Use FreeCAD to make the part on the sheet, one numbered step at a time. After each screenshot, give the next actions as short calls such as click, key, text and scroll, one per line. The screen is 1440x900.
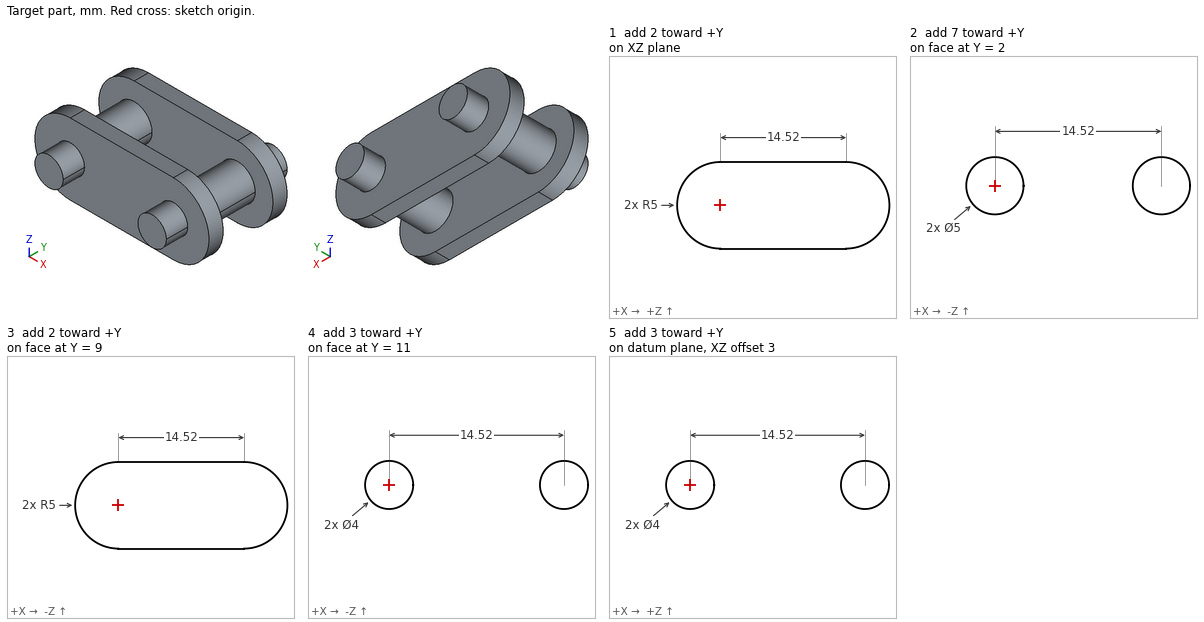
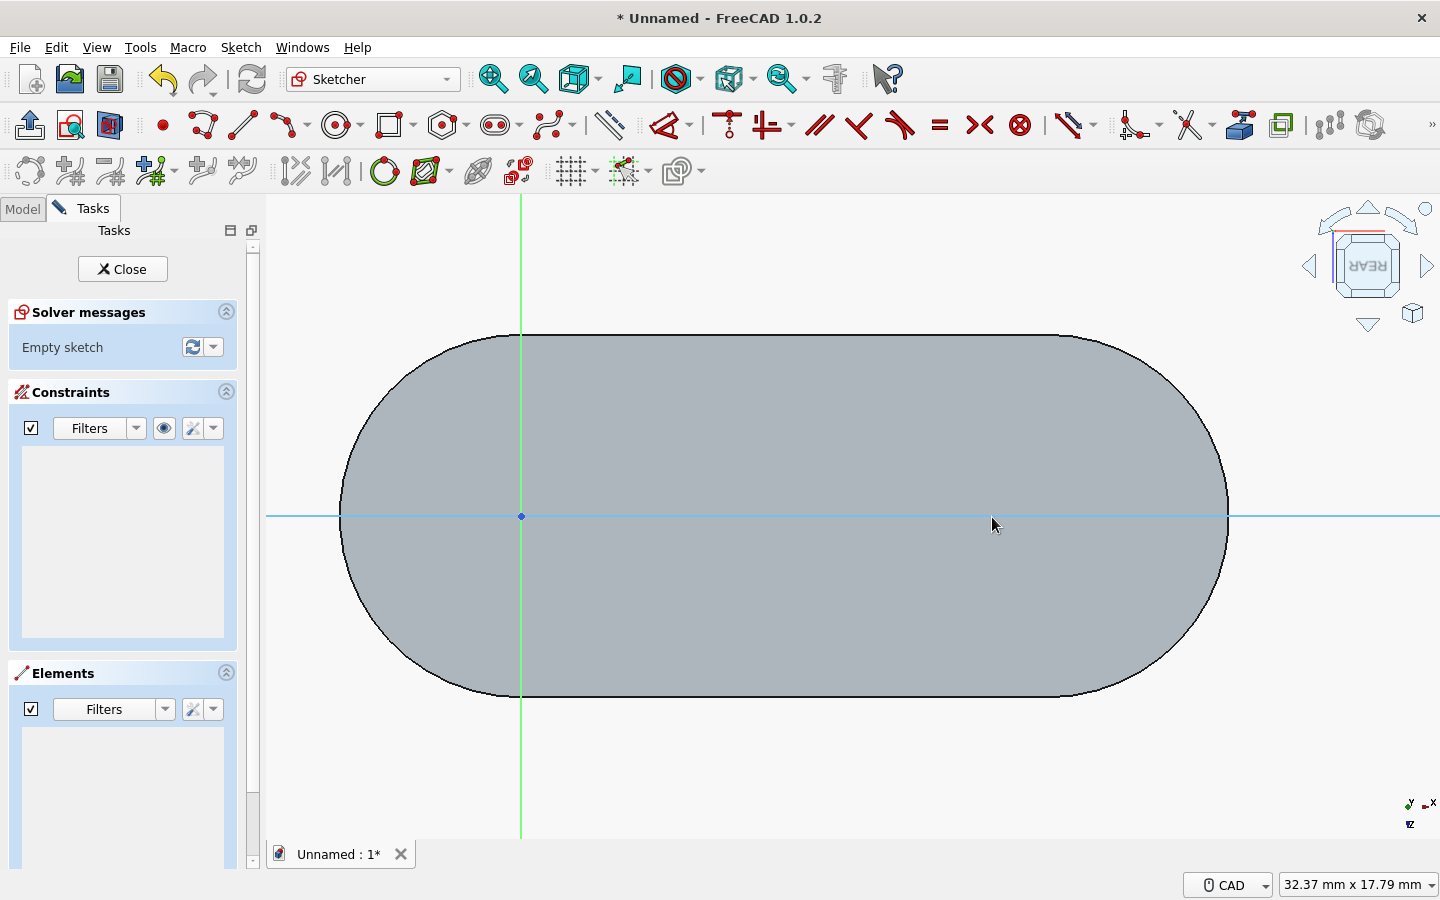
click(336, 126)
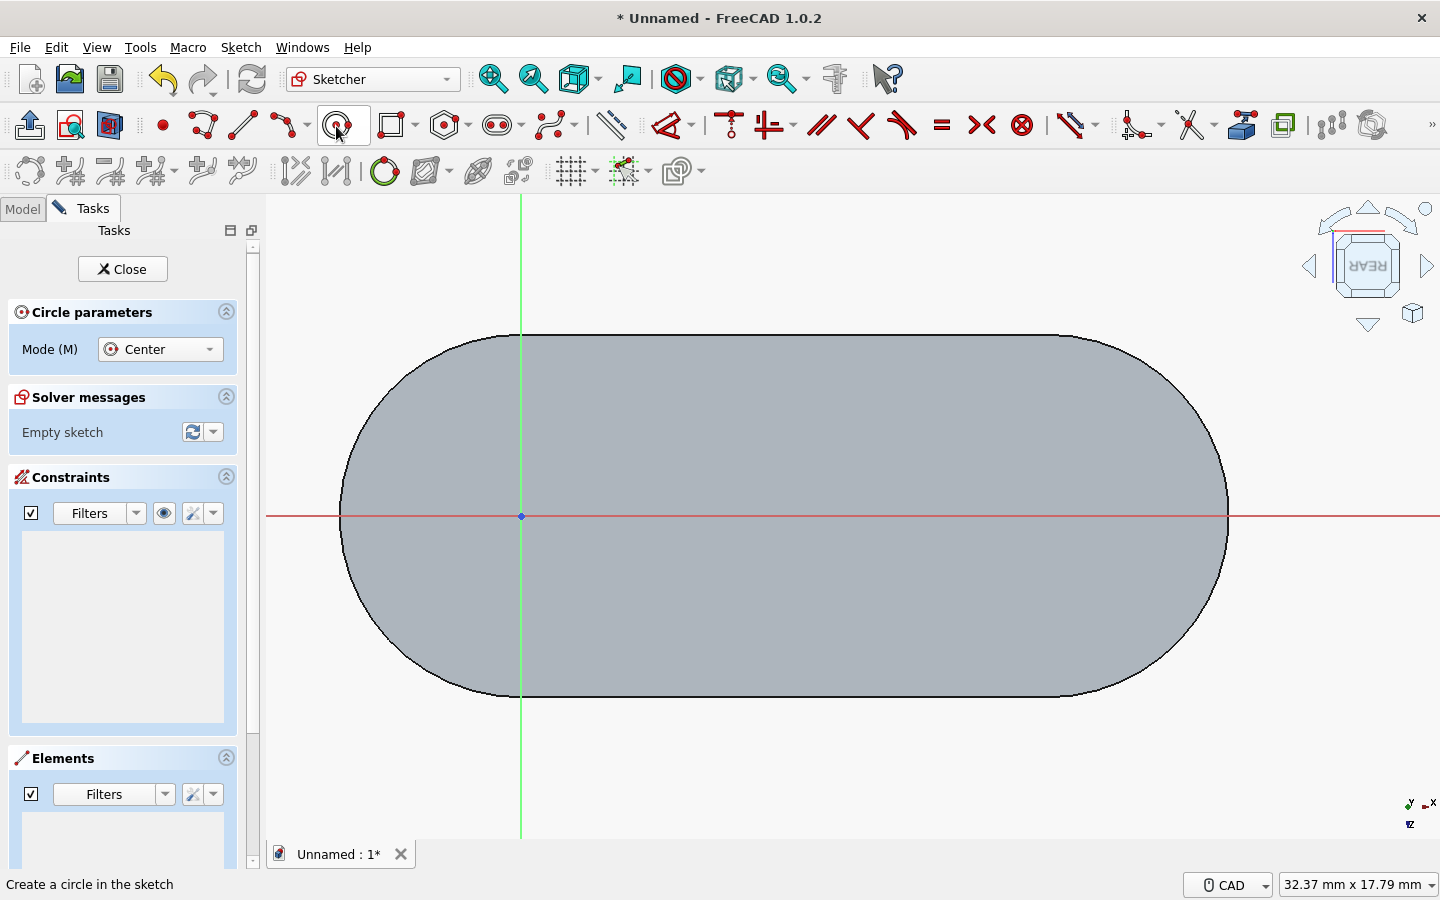
click(521, 516)
move(585, 452)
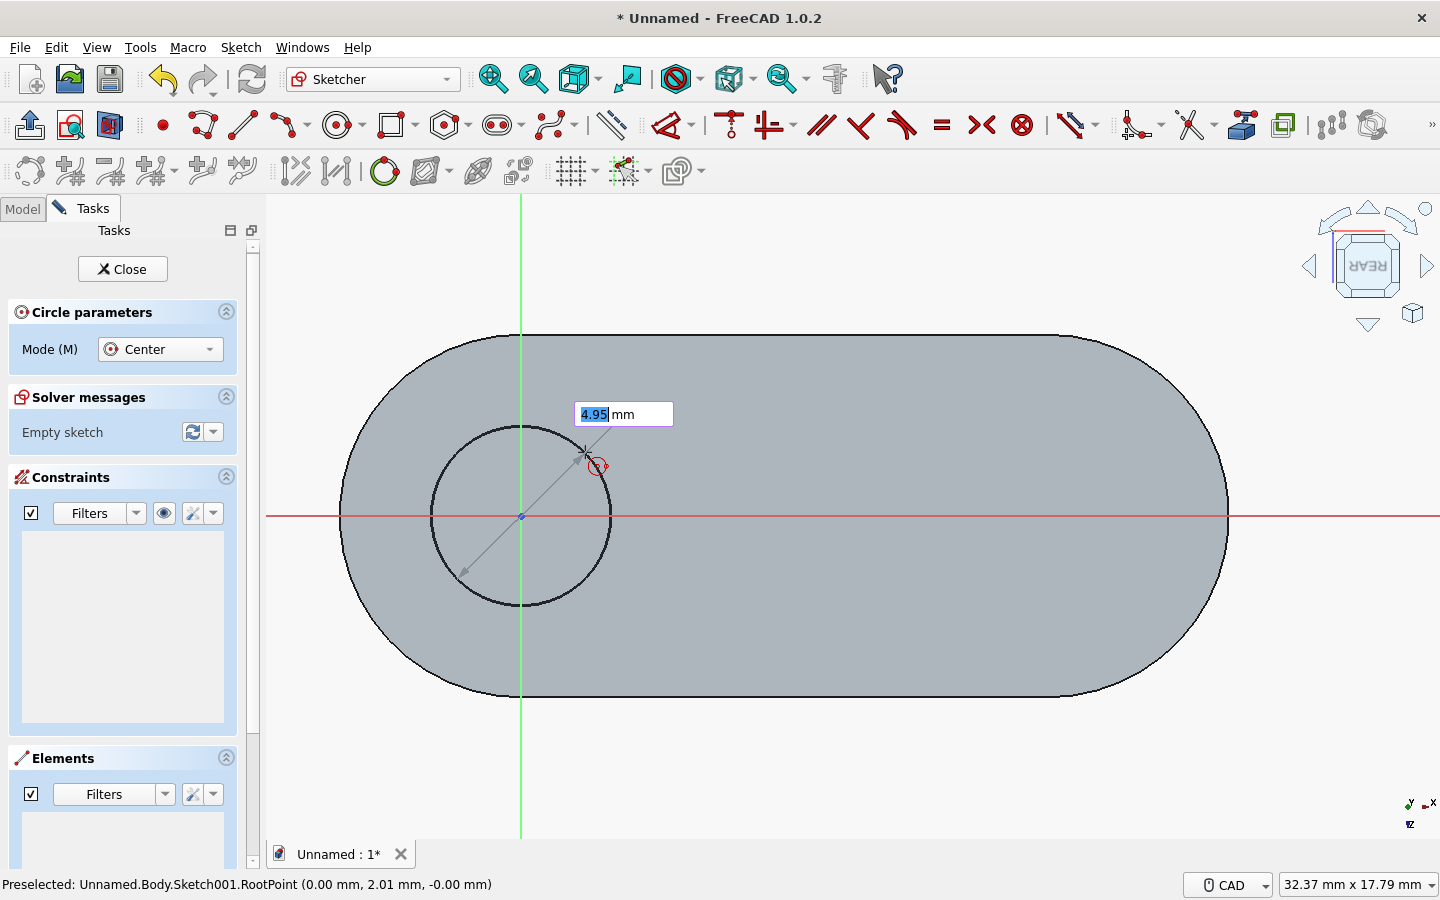
text(5)
key(Return)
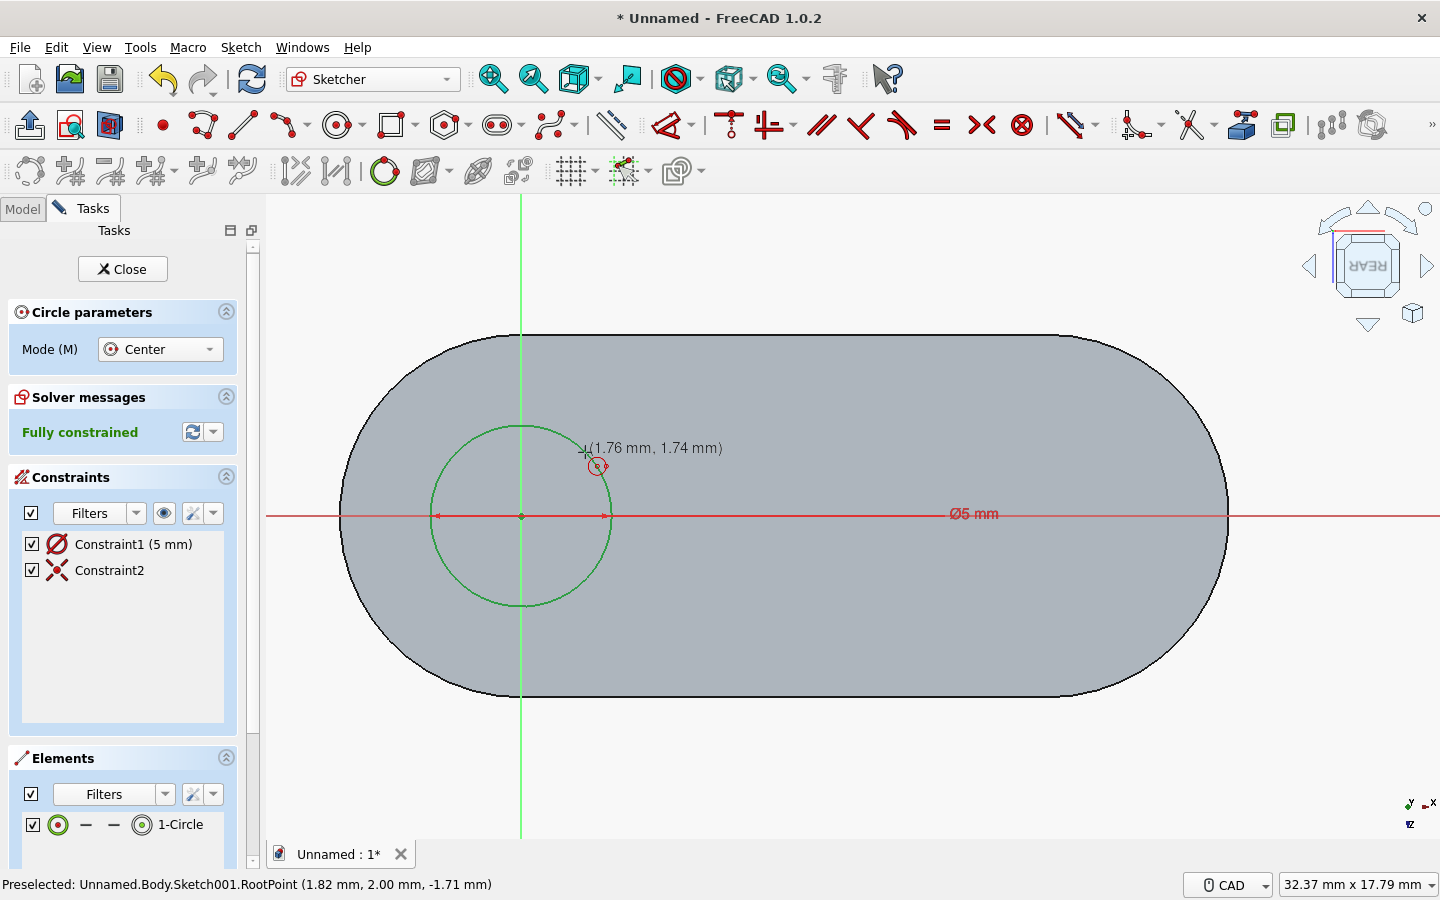
click(1048, 516)
move(1112, 452)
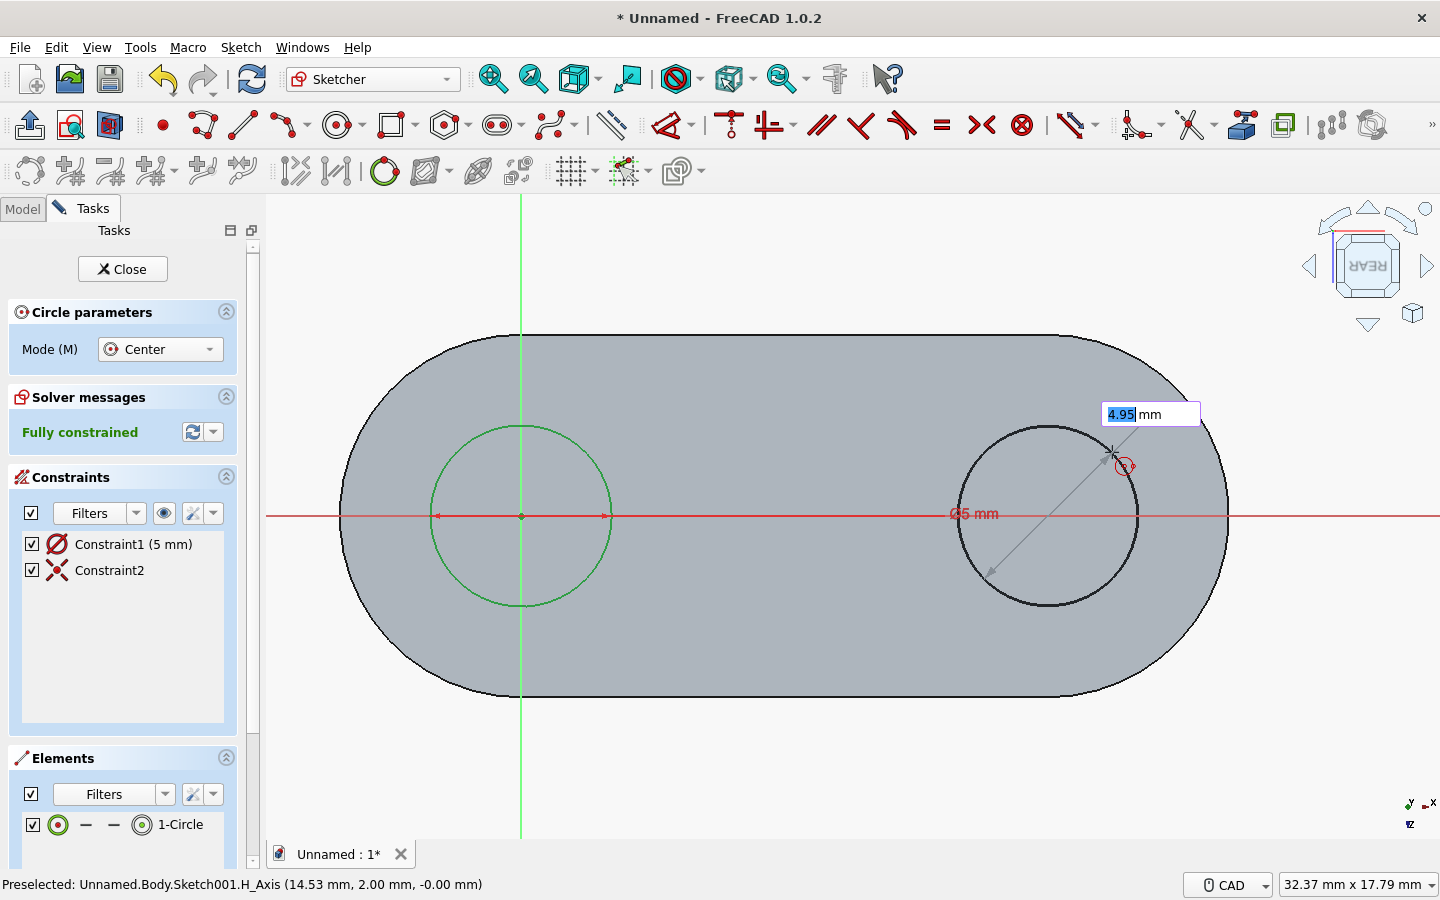
text(5)
key(Return)
key(Escape)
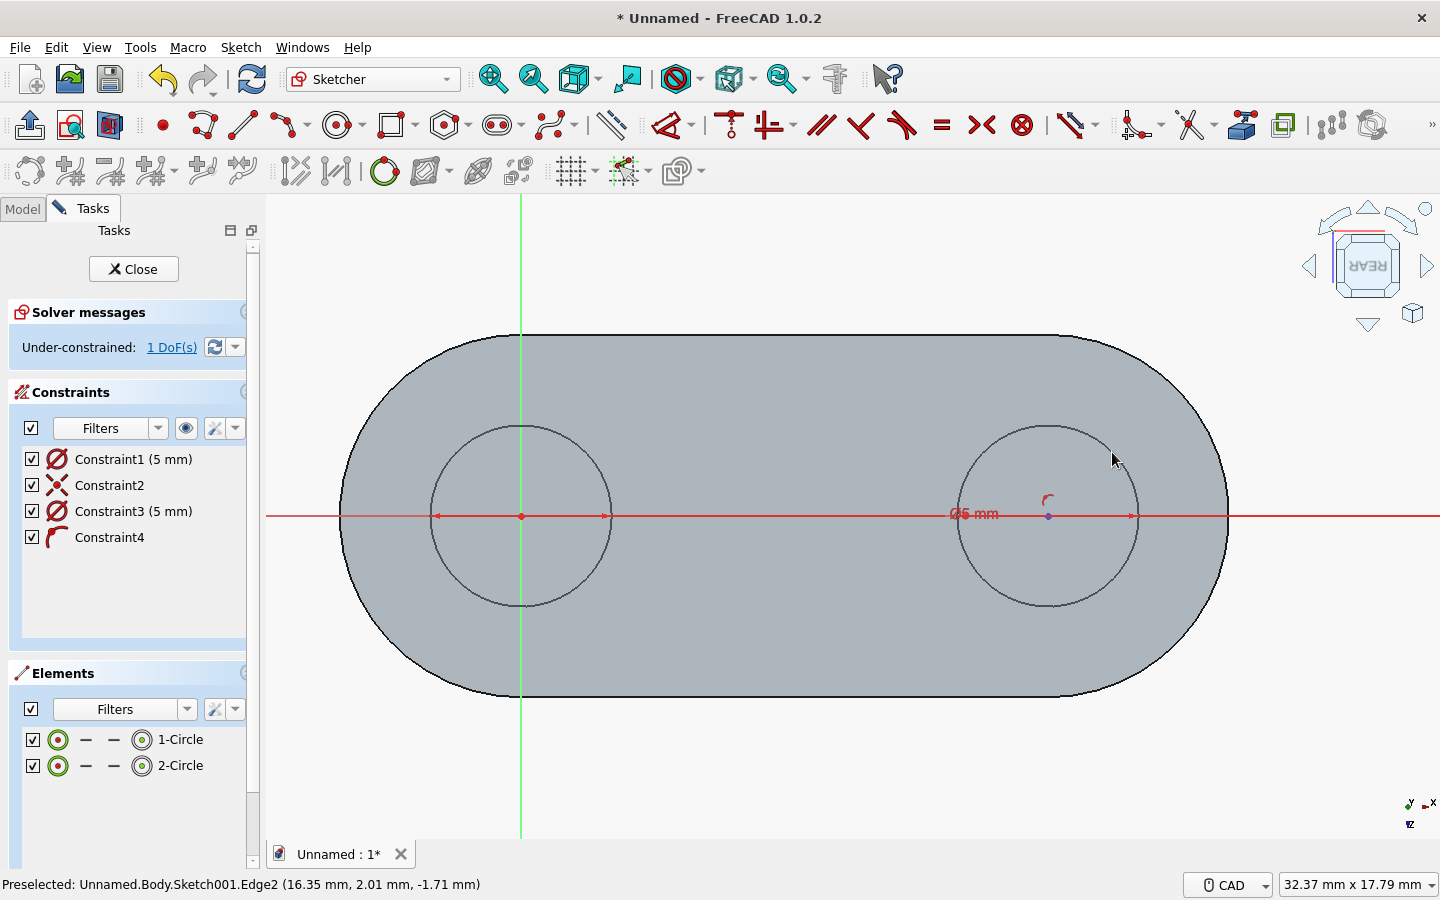
key(d)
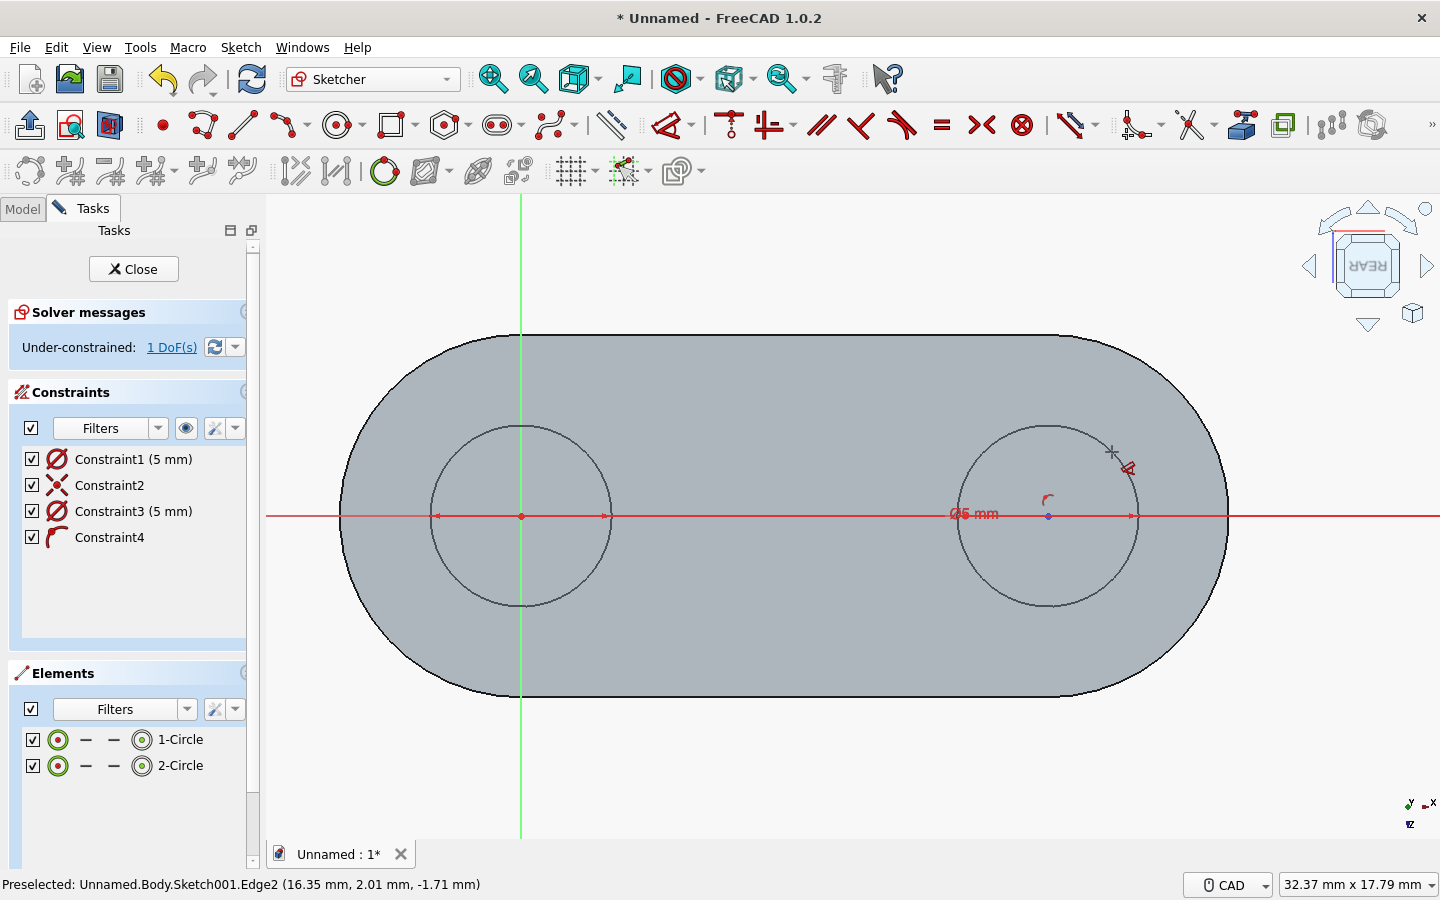
click(1048, 516)
click(785, 550)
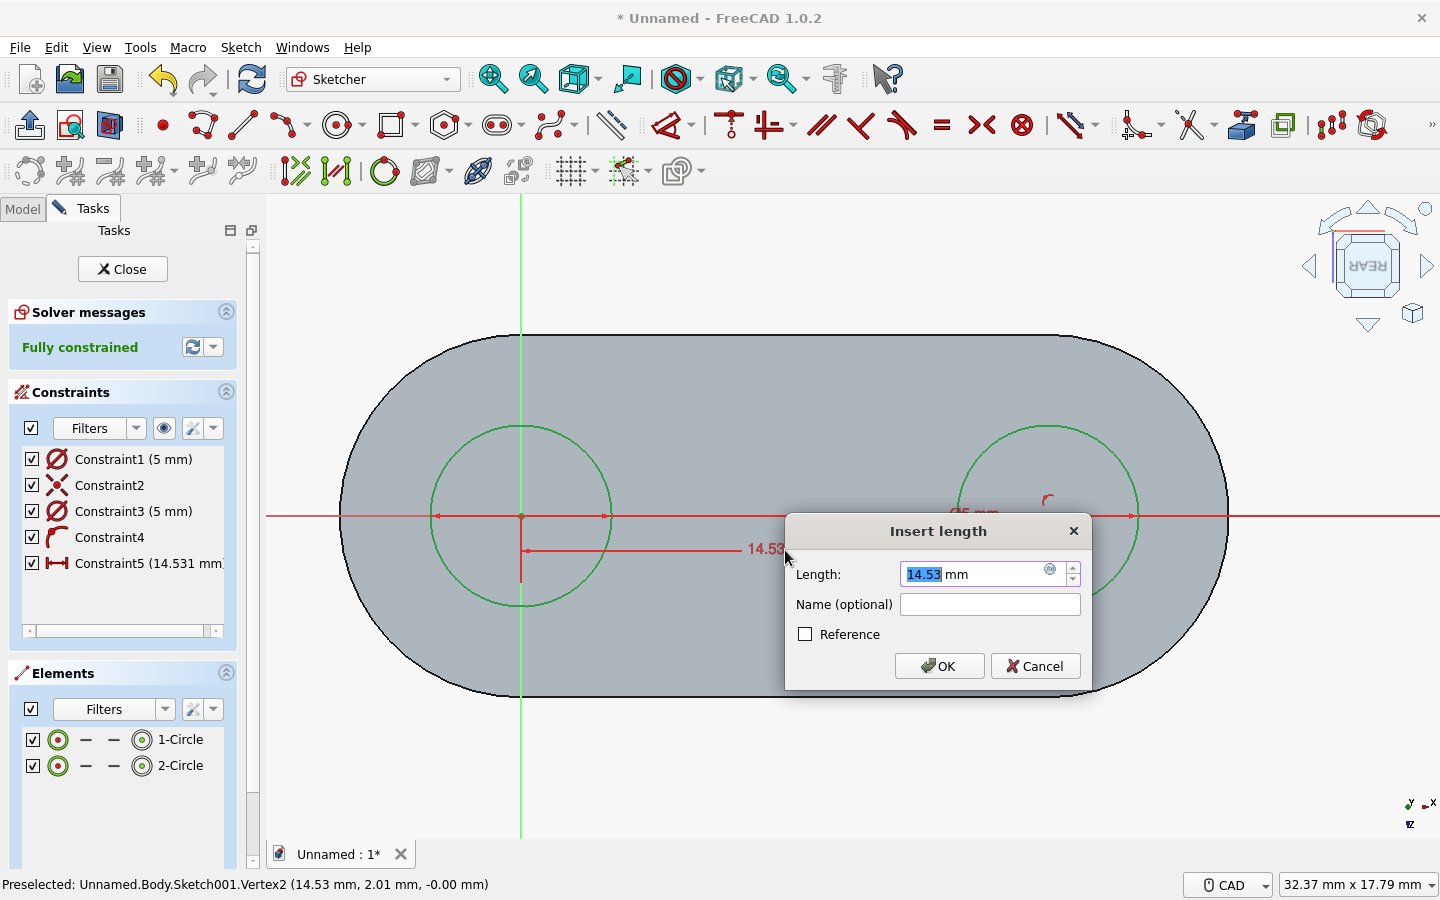
text(14.52)
key(Return)
key(Escape)